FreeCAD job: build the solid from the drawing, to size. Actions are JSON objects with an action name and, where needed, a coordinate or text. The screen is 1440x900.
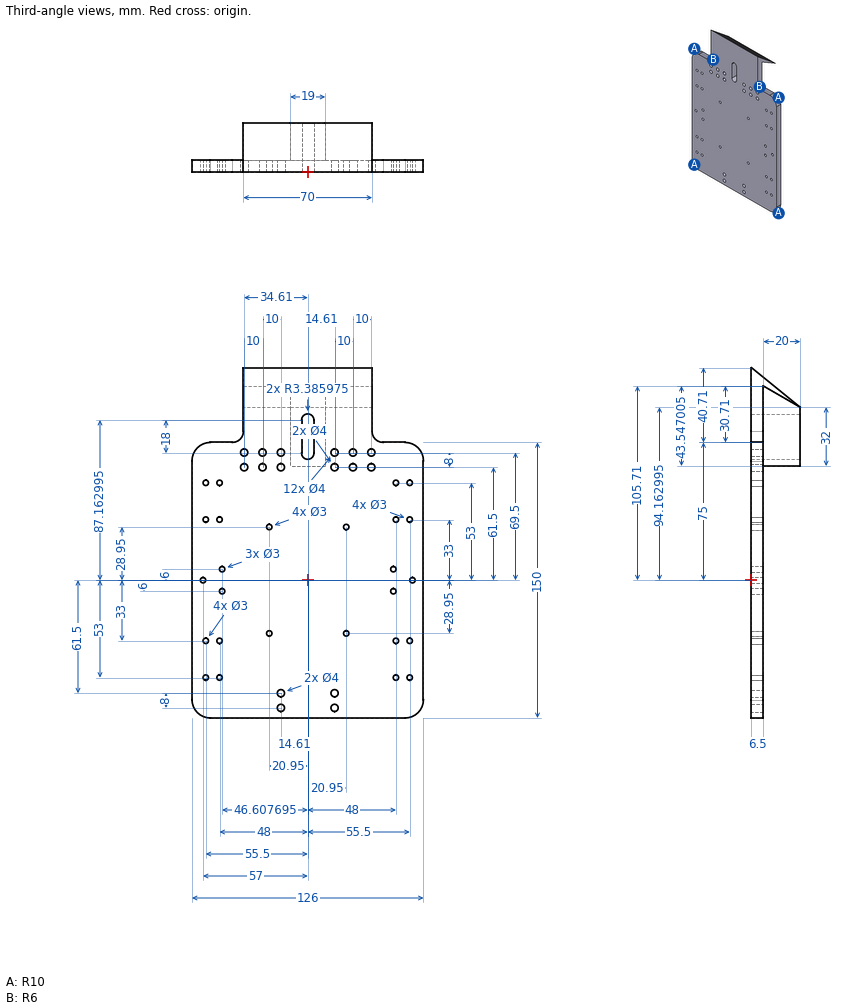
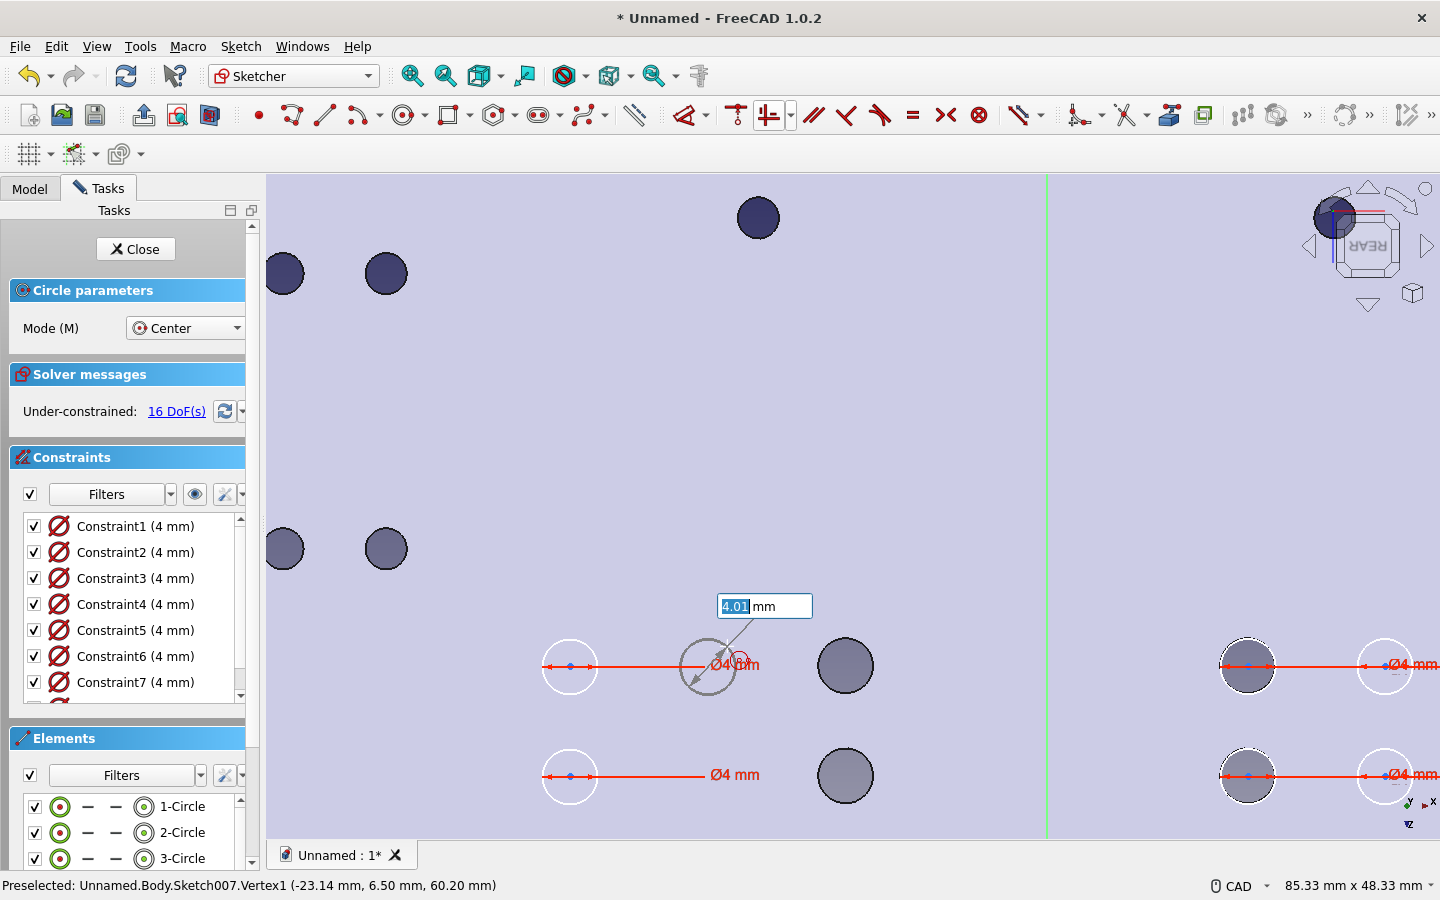
{"action": "type", "text": "4"}
{"action": "key", "text": "Return"}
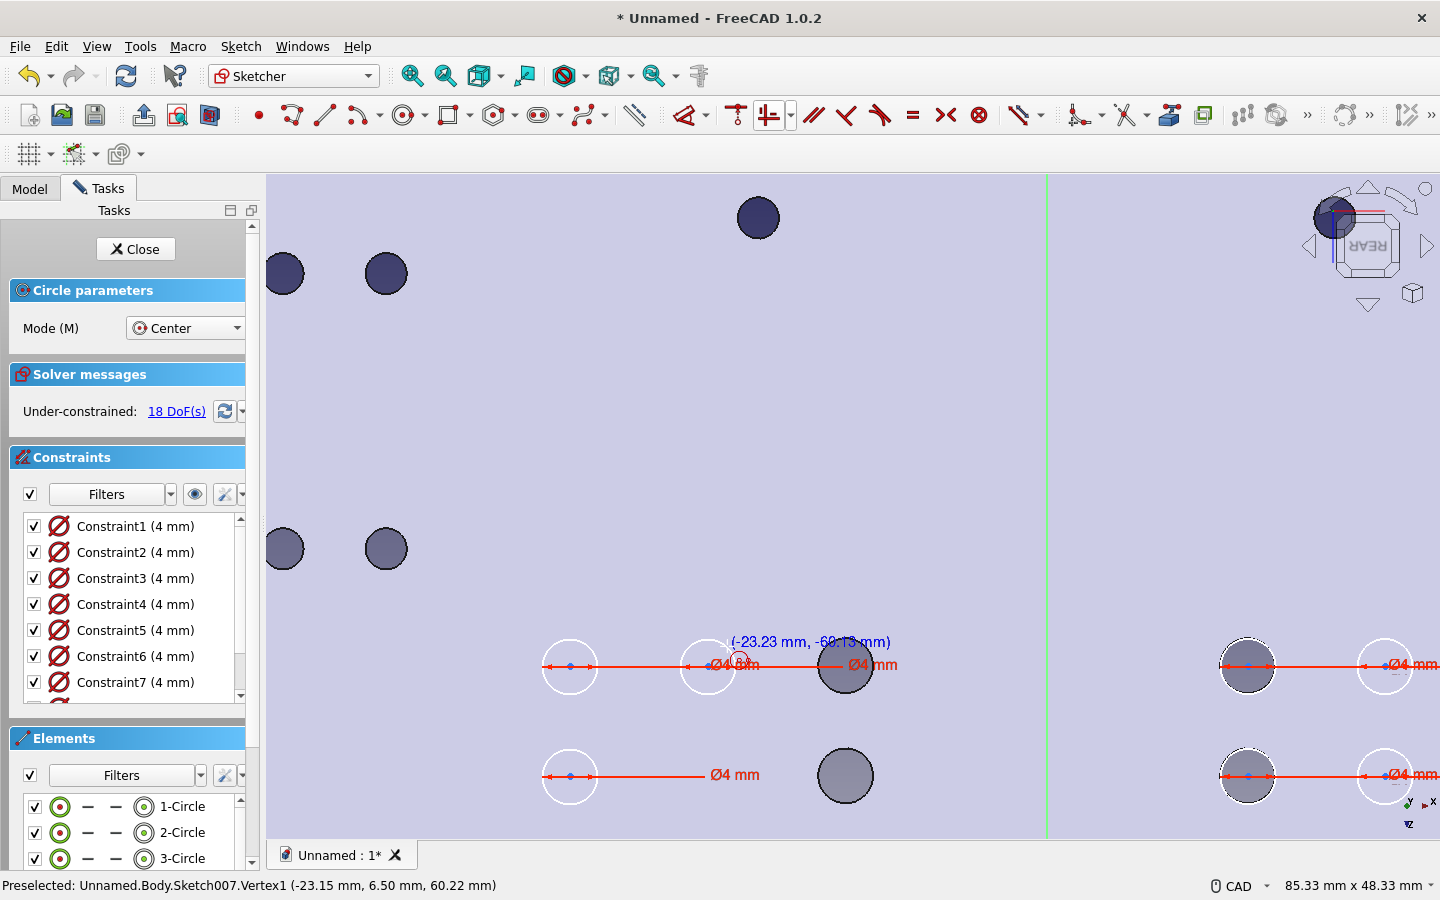
{"action": "left_click", "coordinate": [708, 776]}
{"action": "mouse_move", "coordinate": [727, 756]}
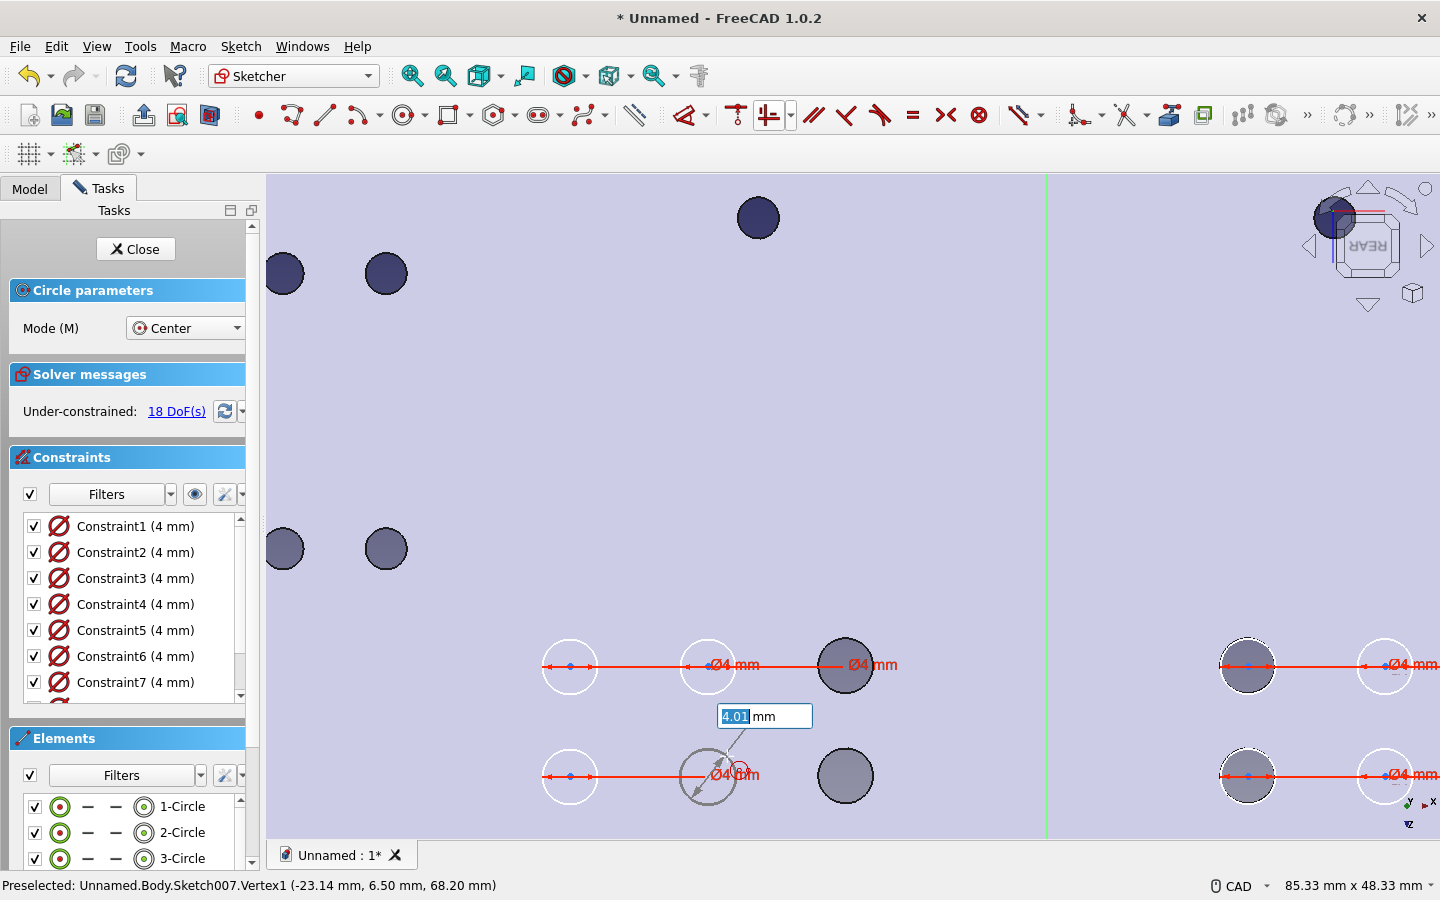
{"action": "type", "text": "4"}
{"action": "key", "text": "Return"}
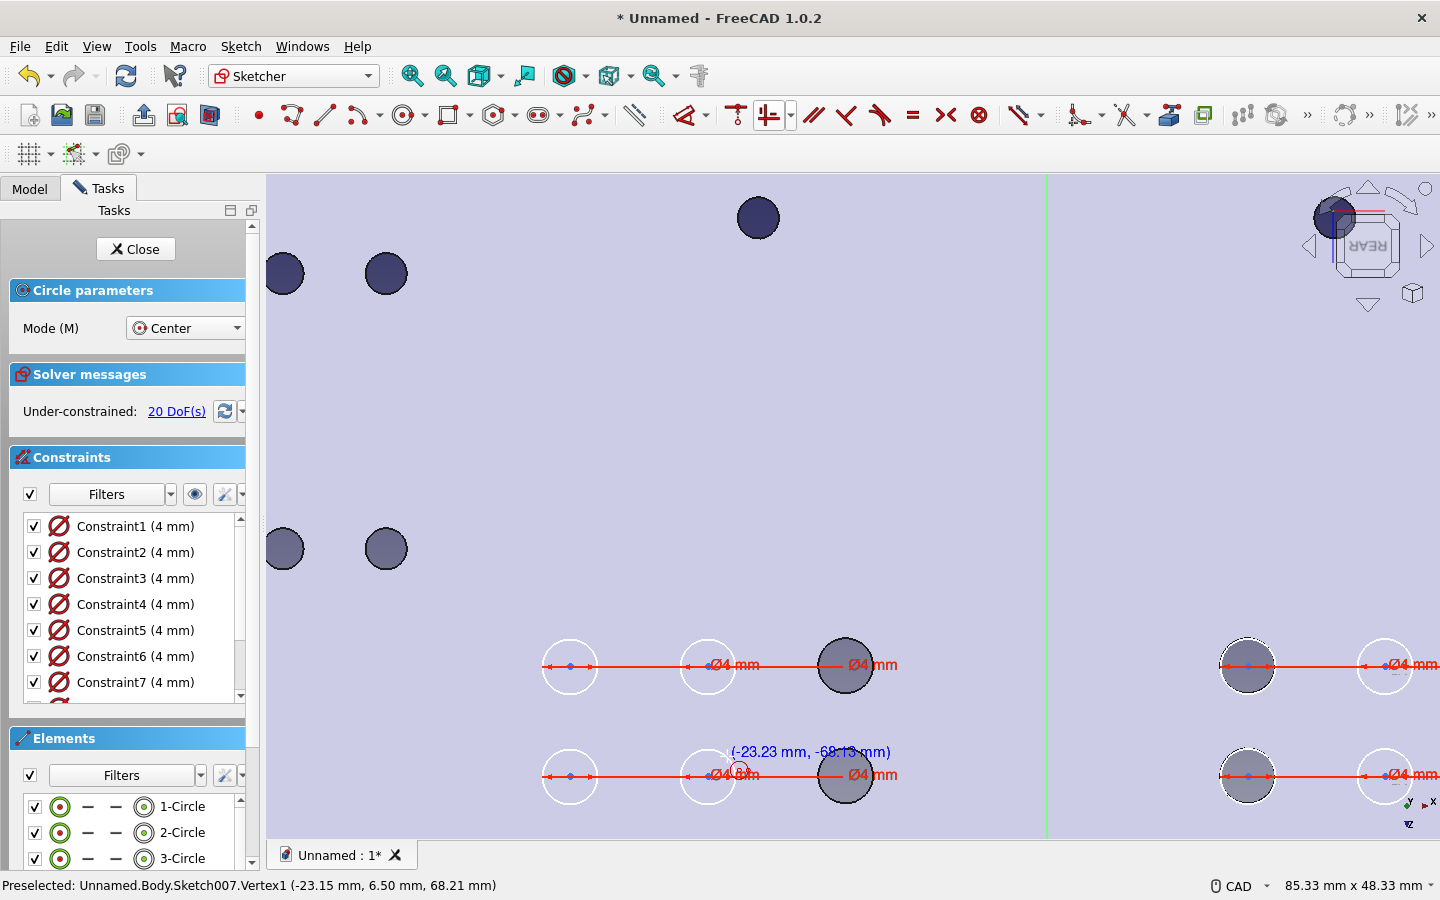
{"action": "left_click", "coordinate": [846, 666]}
{"action": "mouse_move", "coordinate": [865, 646]}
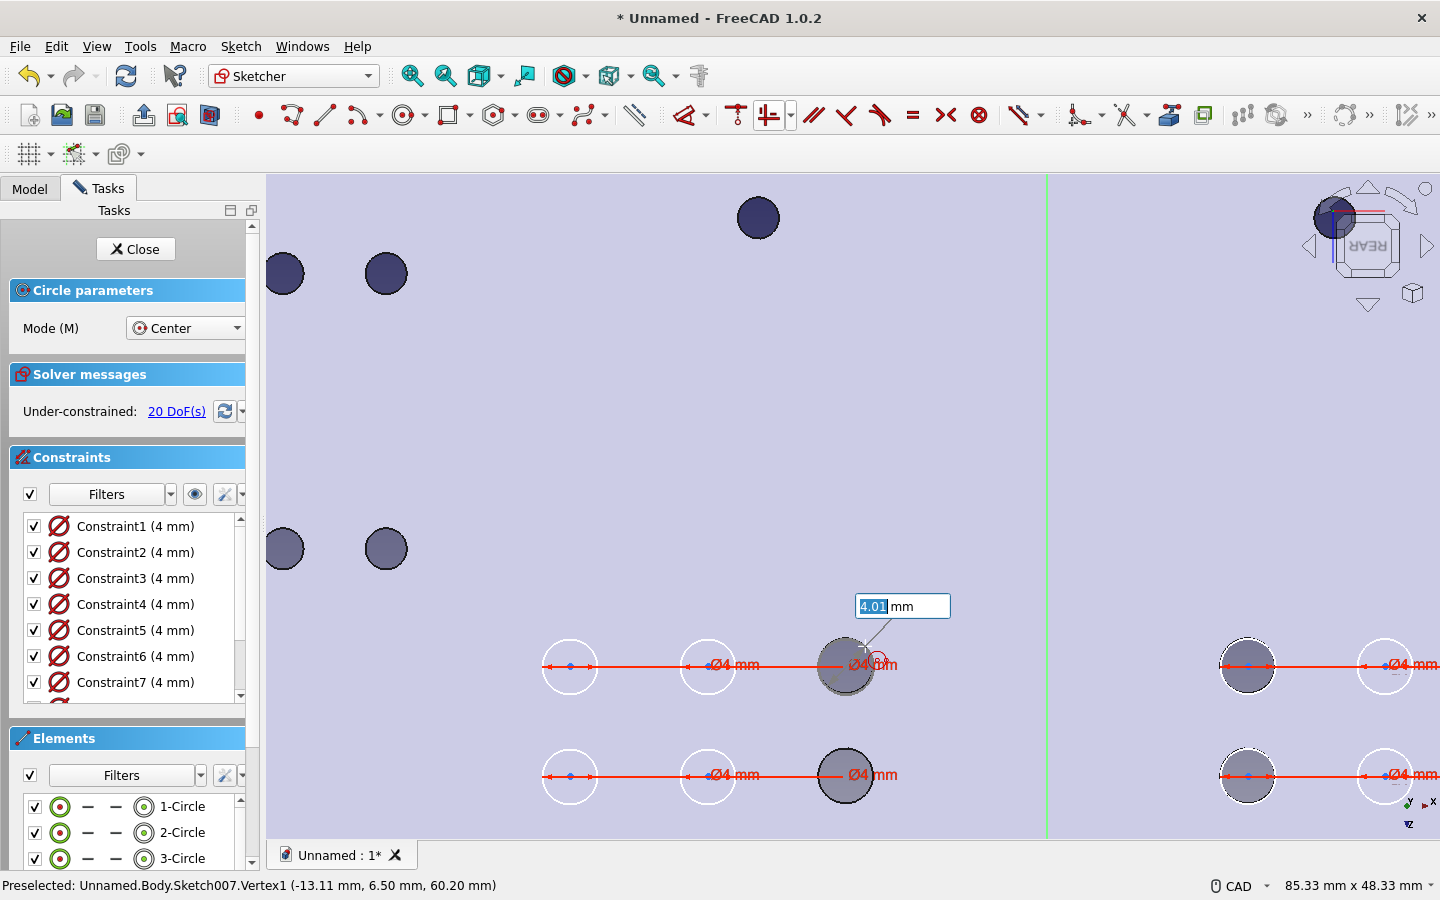
{"action": "type", "text": "4"}
{"action": "key", "text": "Return"}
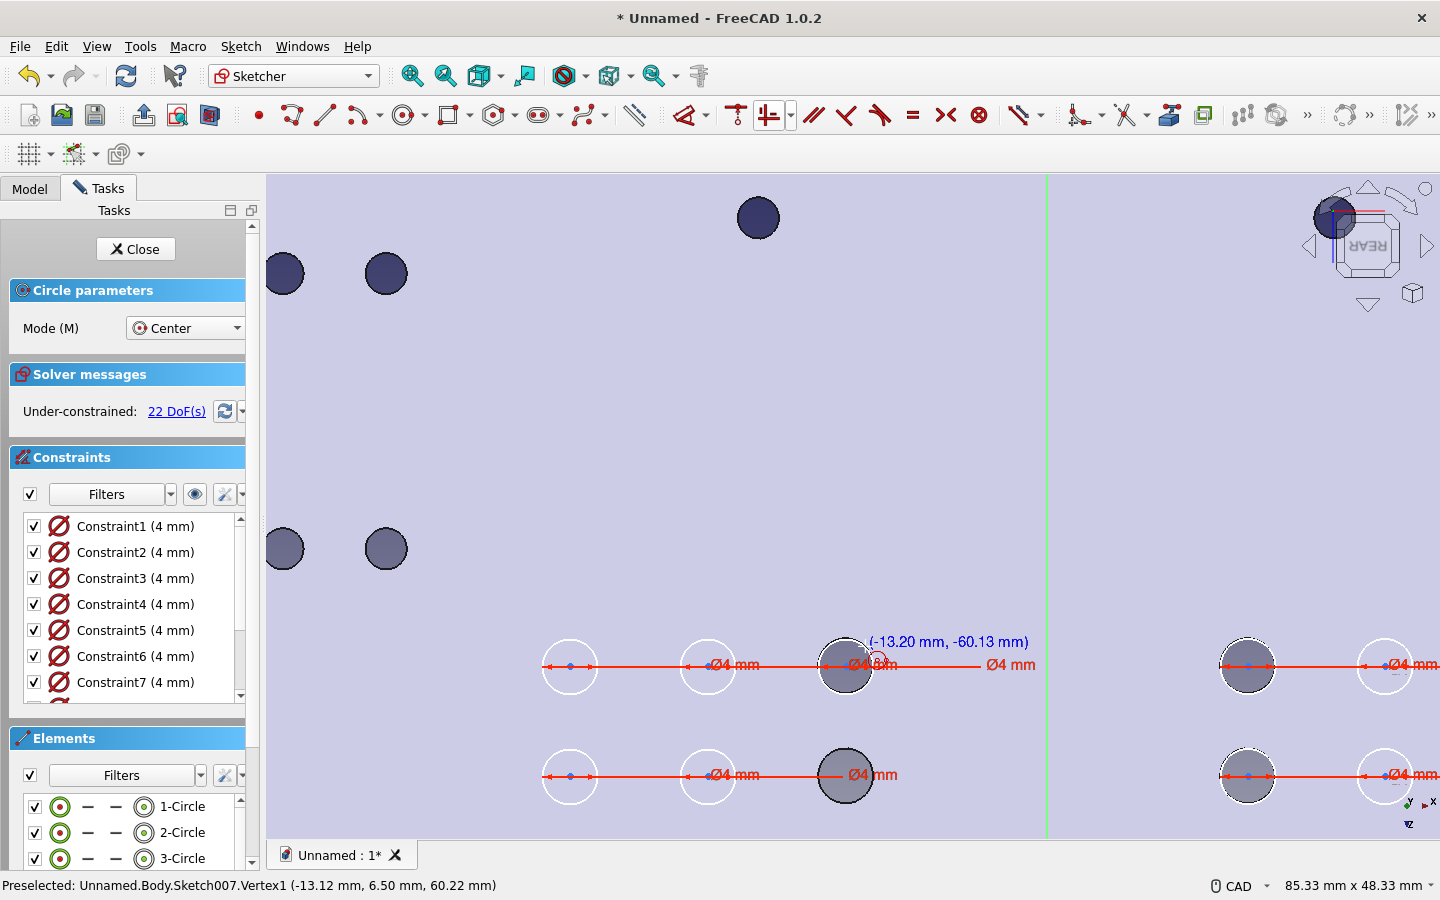
{"action": "left_click", "coordinate": [846, 776]}
{"action": "mouse_move", "coordinate": [865, 756]}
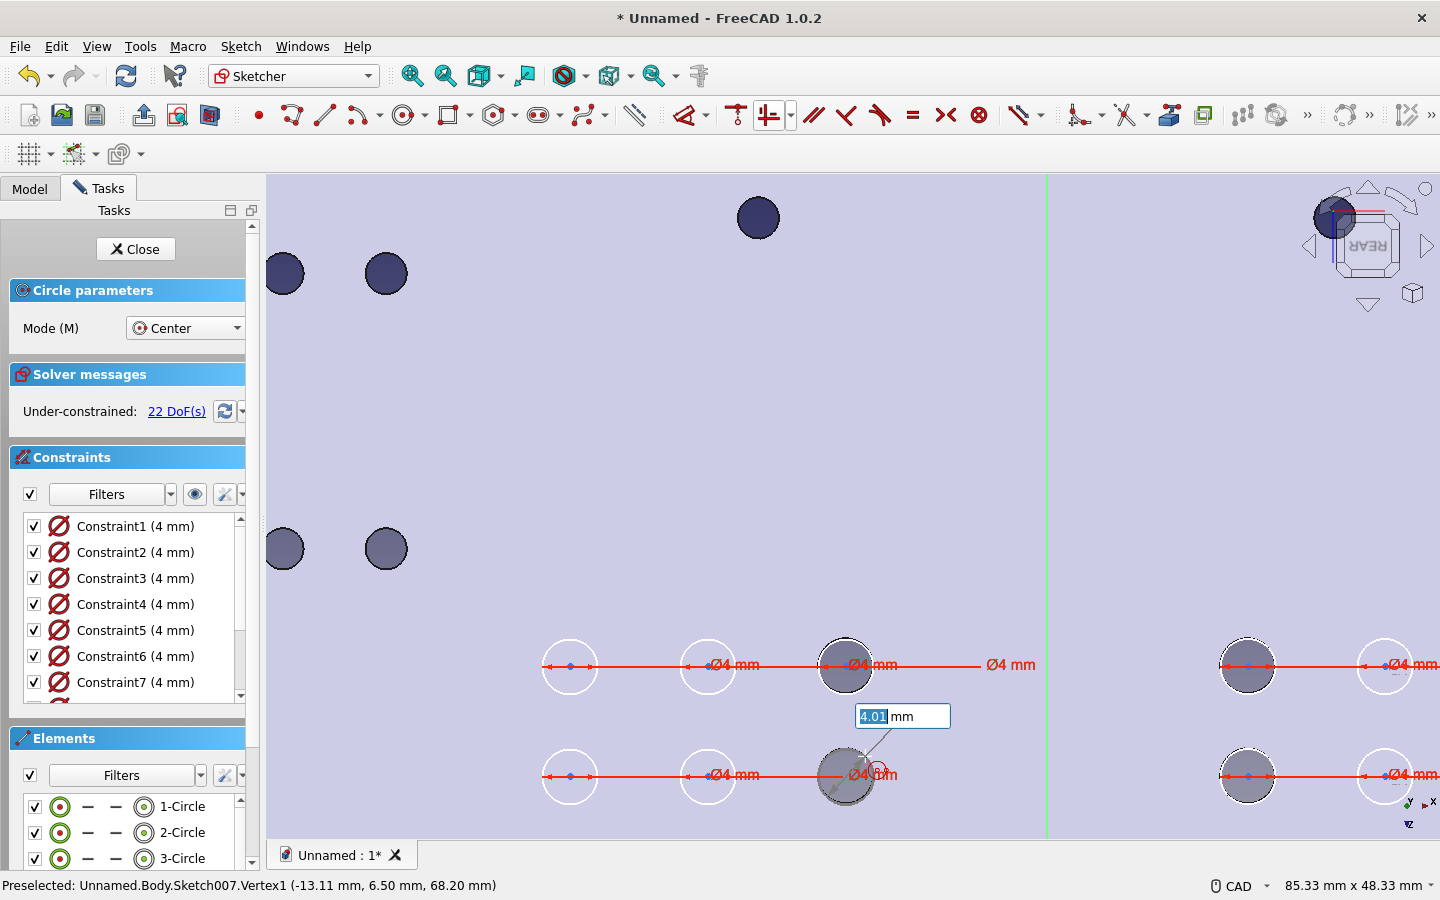
{"action": "type", "text": "4"}
{"action": "key", "text": "Return"}
{"action": "key", "text": "Escape"}